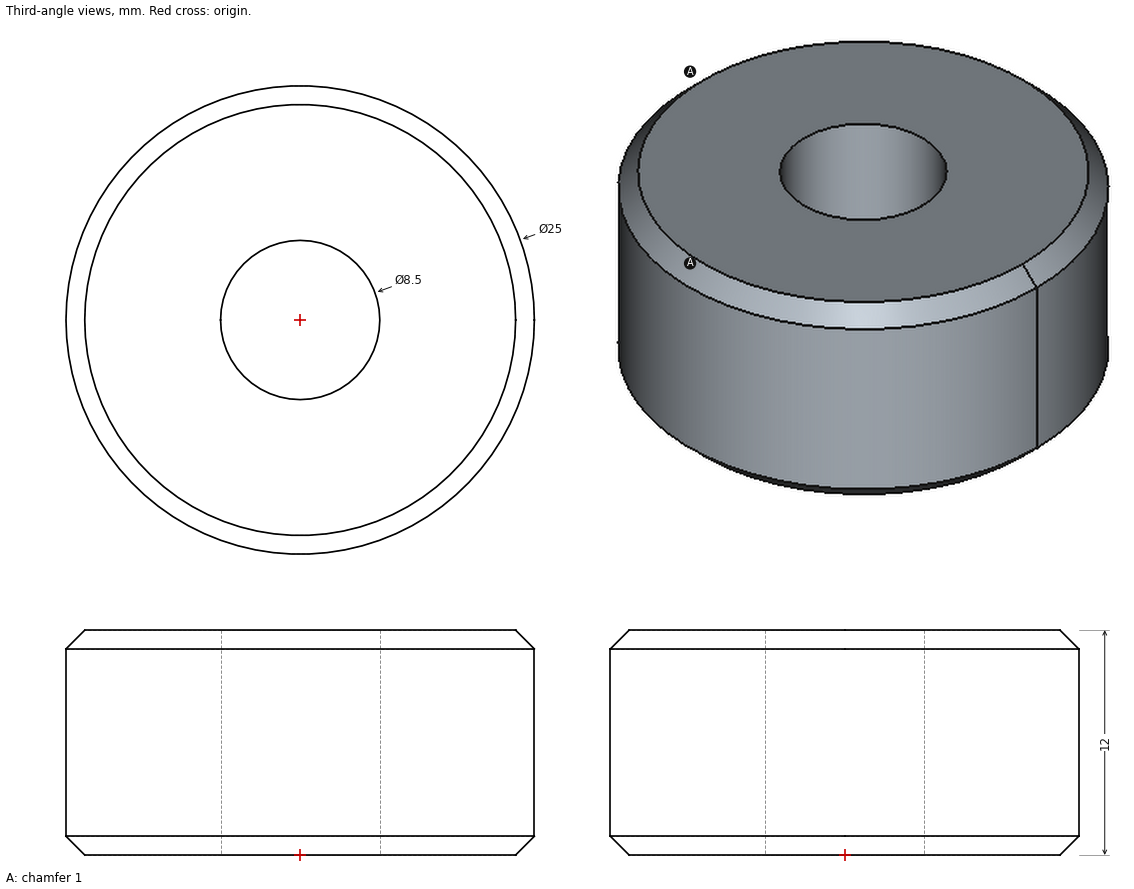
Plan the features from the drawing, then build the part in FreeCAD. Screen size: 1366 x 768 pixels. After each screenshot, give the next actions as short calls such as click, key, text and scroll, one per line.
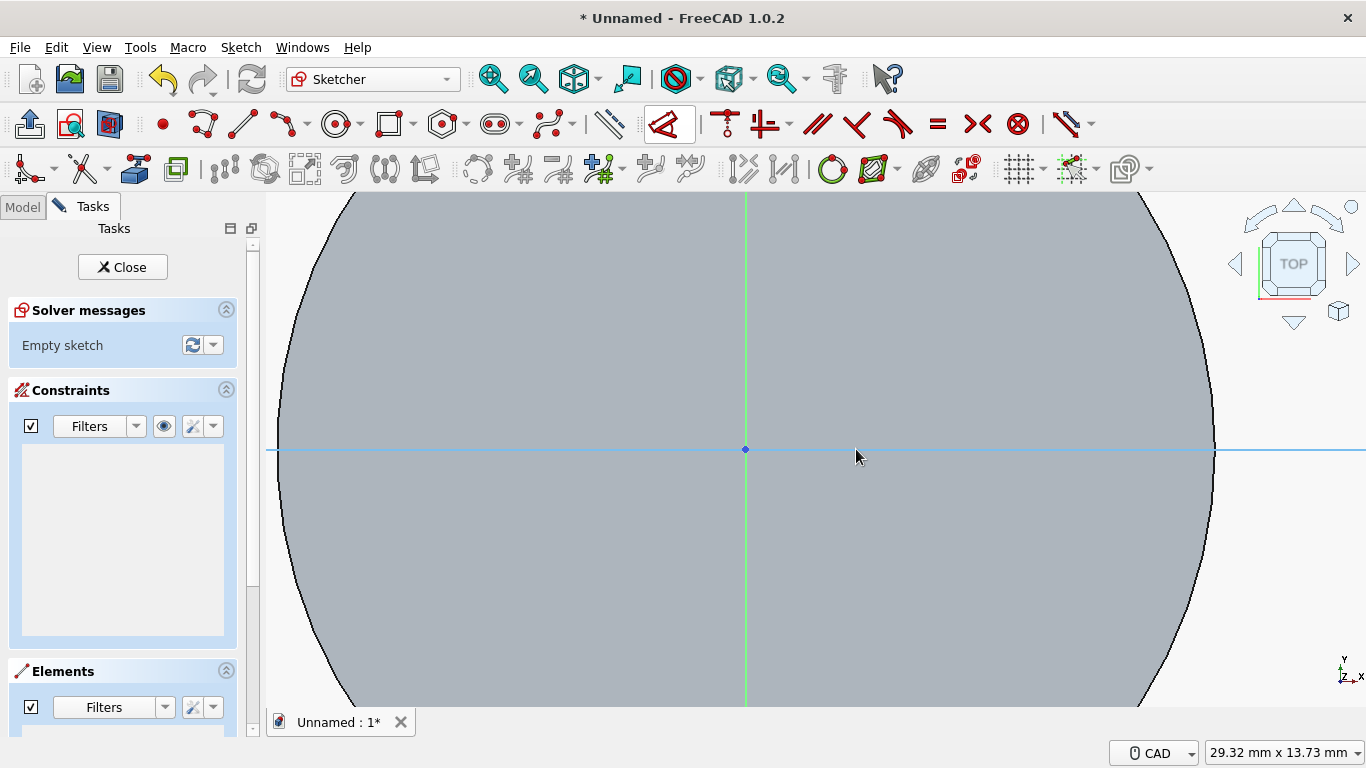
click(336, 124)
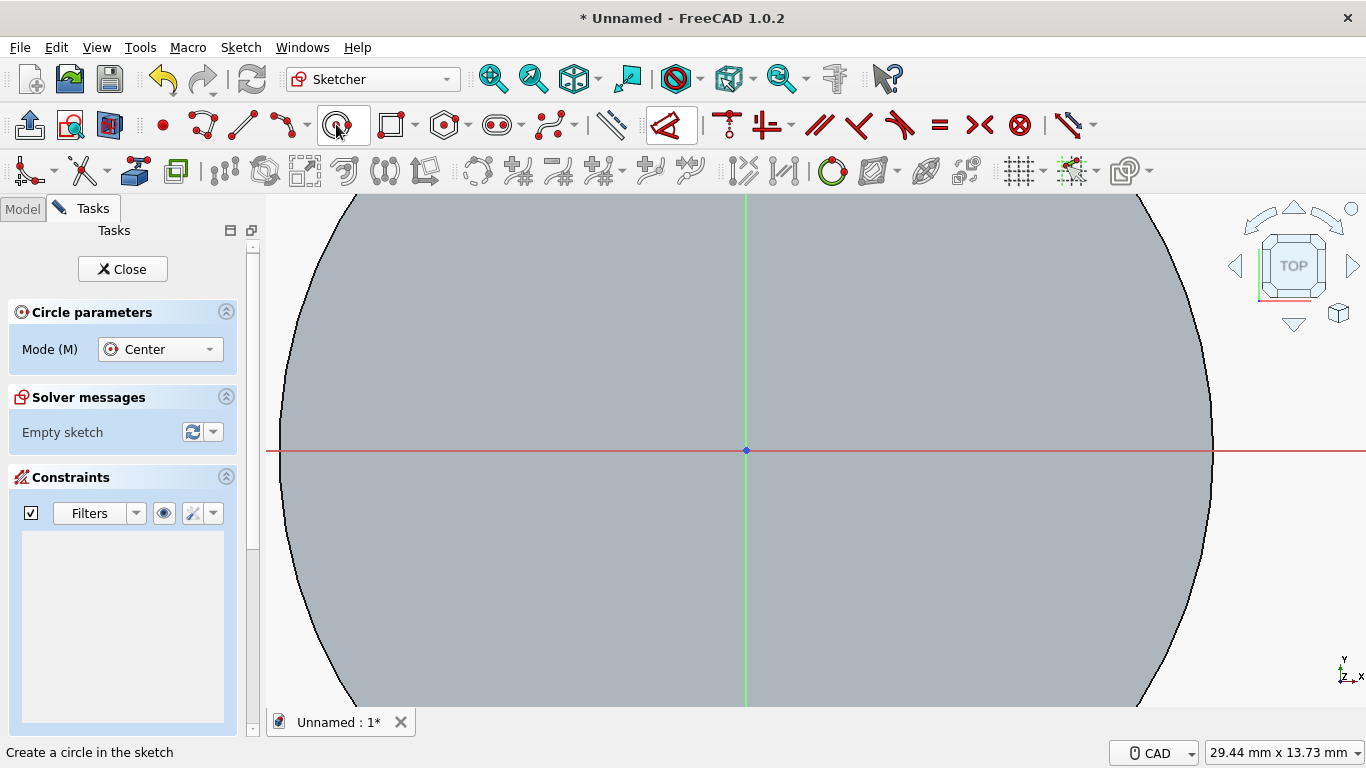
click(746, 450)
click(859, 338)
key(Escape)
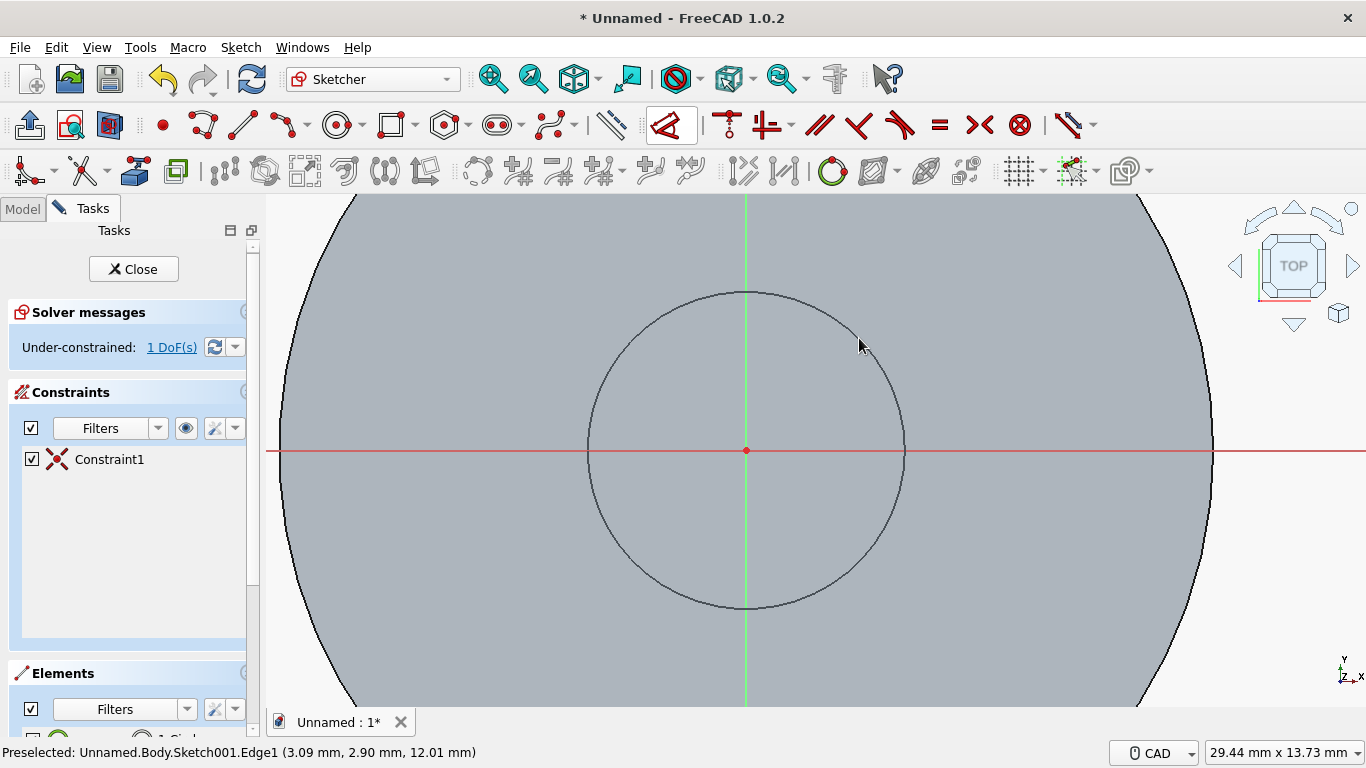
key(d)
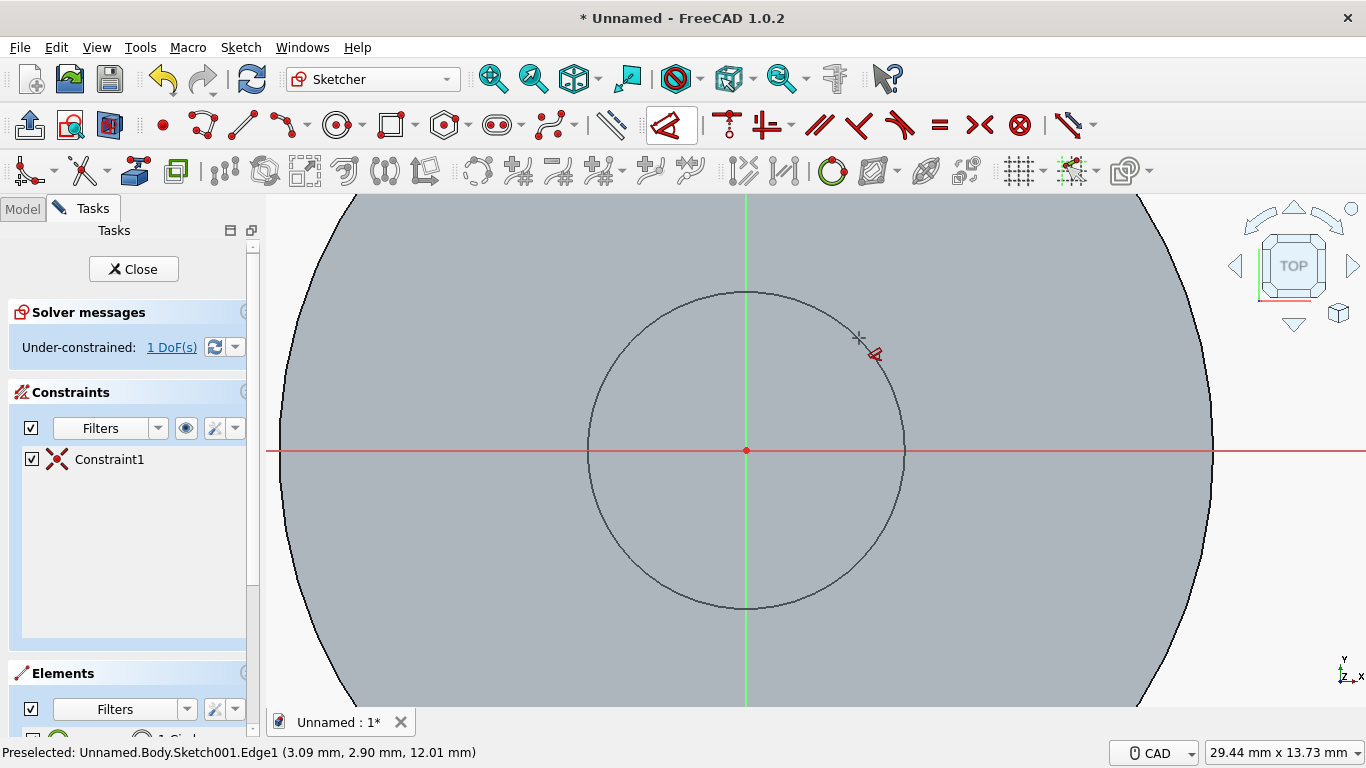
click(858, 338)
click(881, 315)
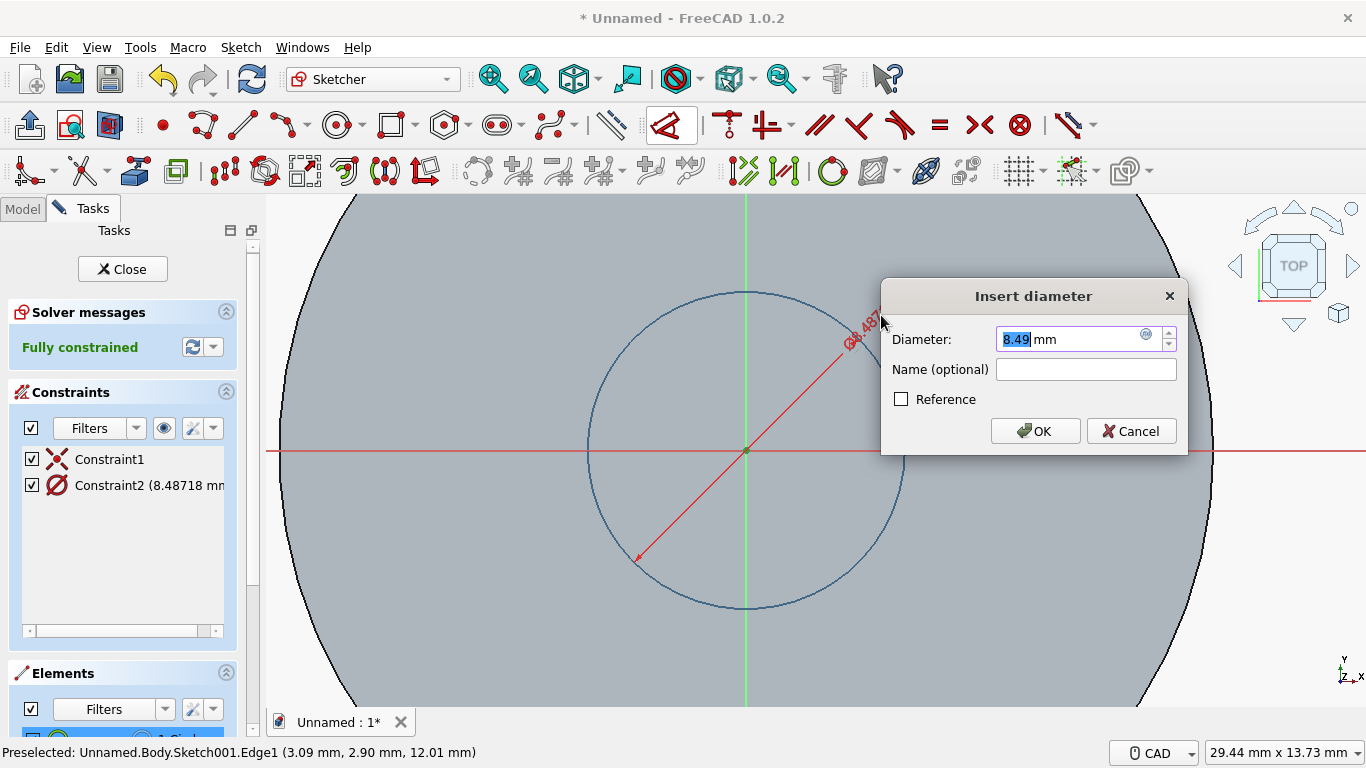
text(8.5)
key(Return)
key(Escape)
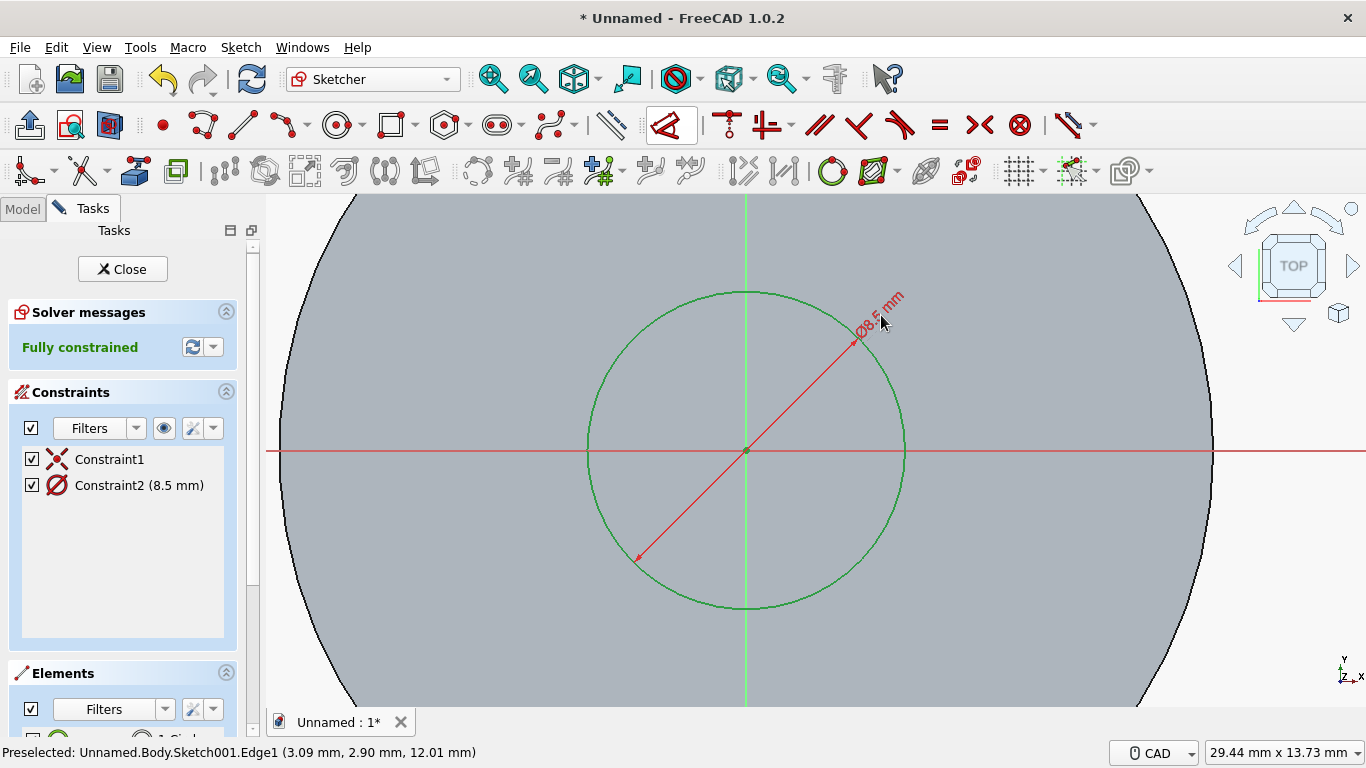
click(123, 269)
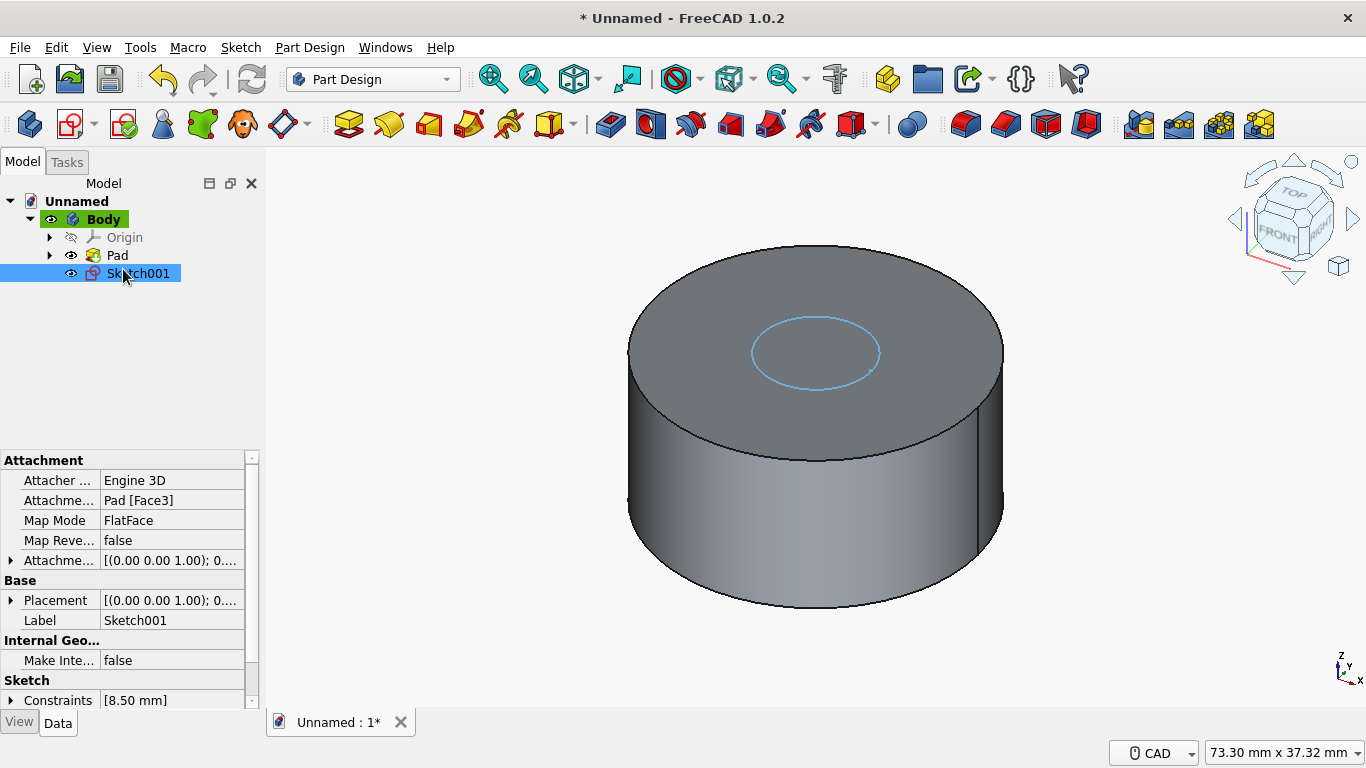
click(612, 124)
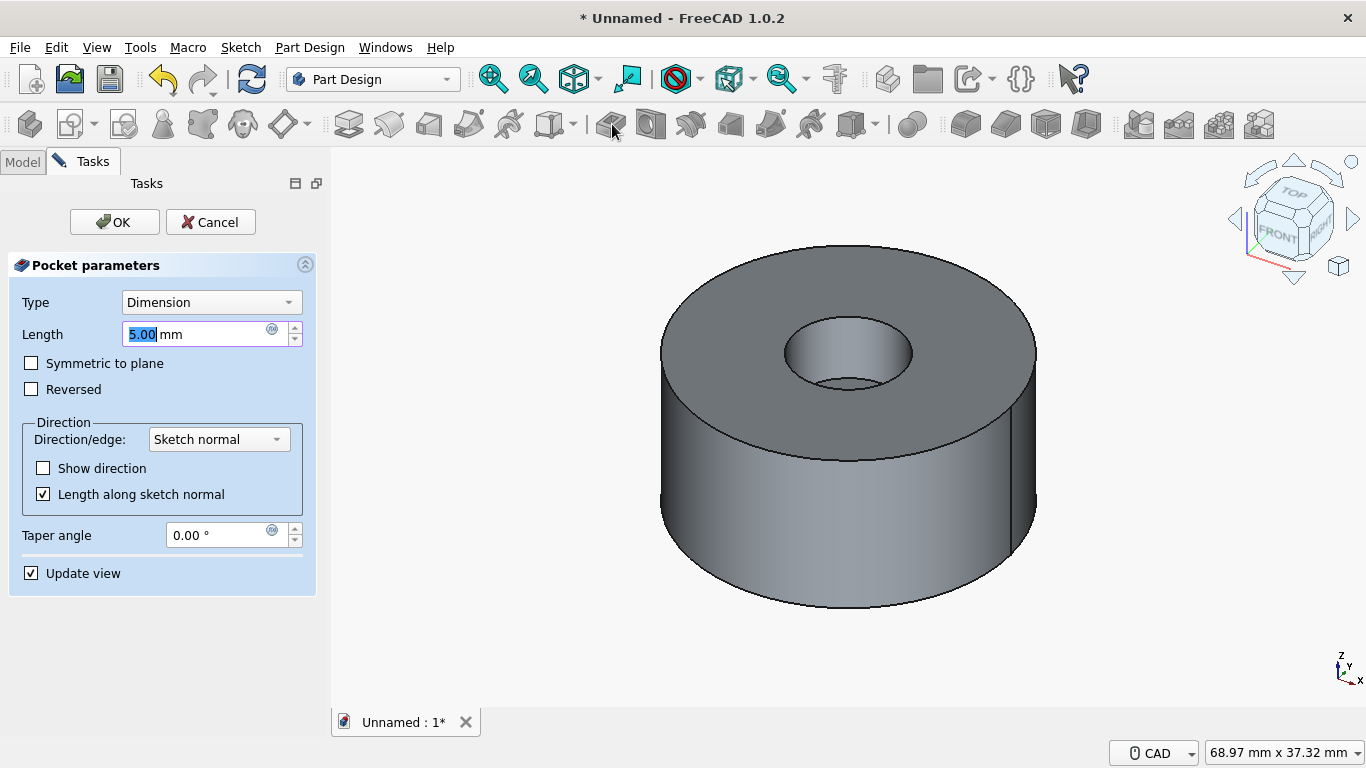
click(212, 302)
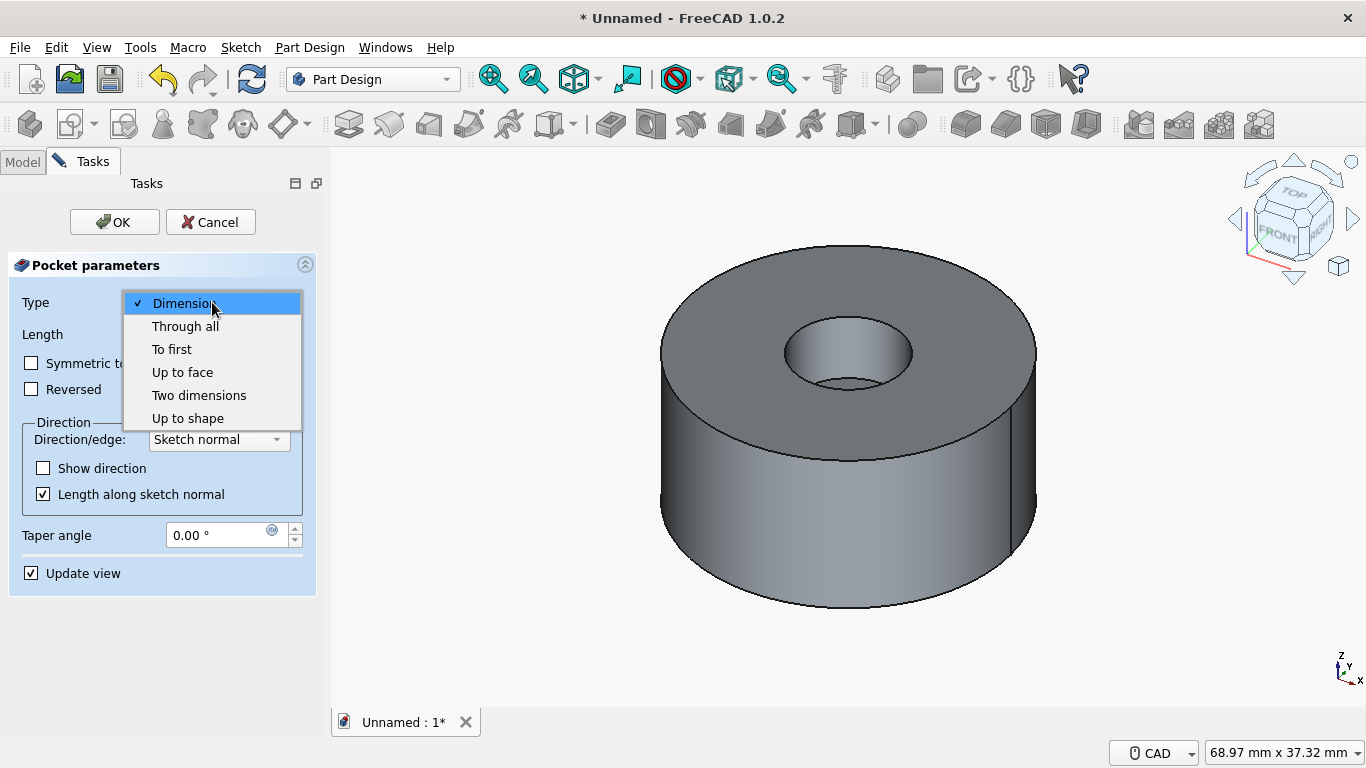
click(212, 326)